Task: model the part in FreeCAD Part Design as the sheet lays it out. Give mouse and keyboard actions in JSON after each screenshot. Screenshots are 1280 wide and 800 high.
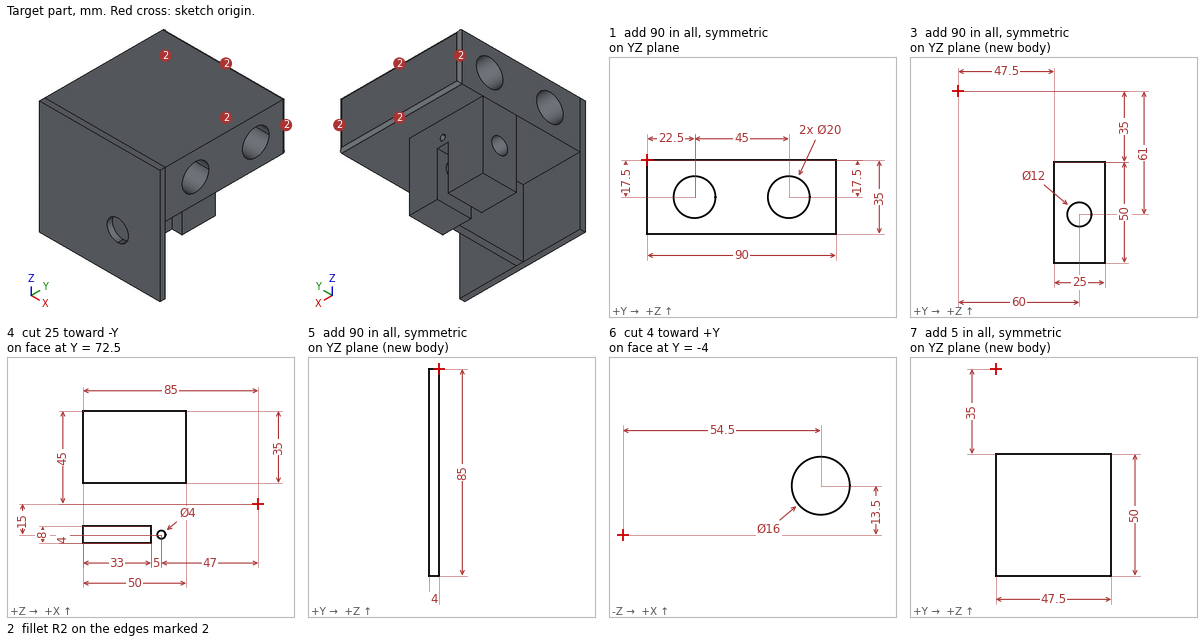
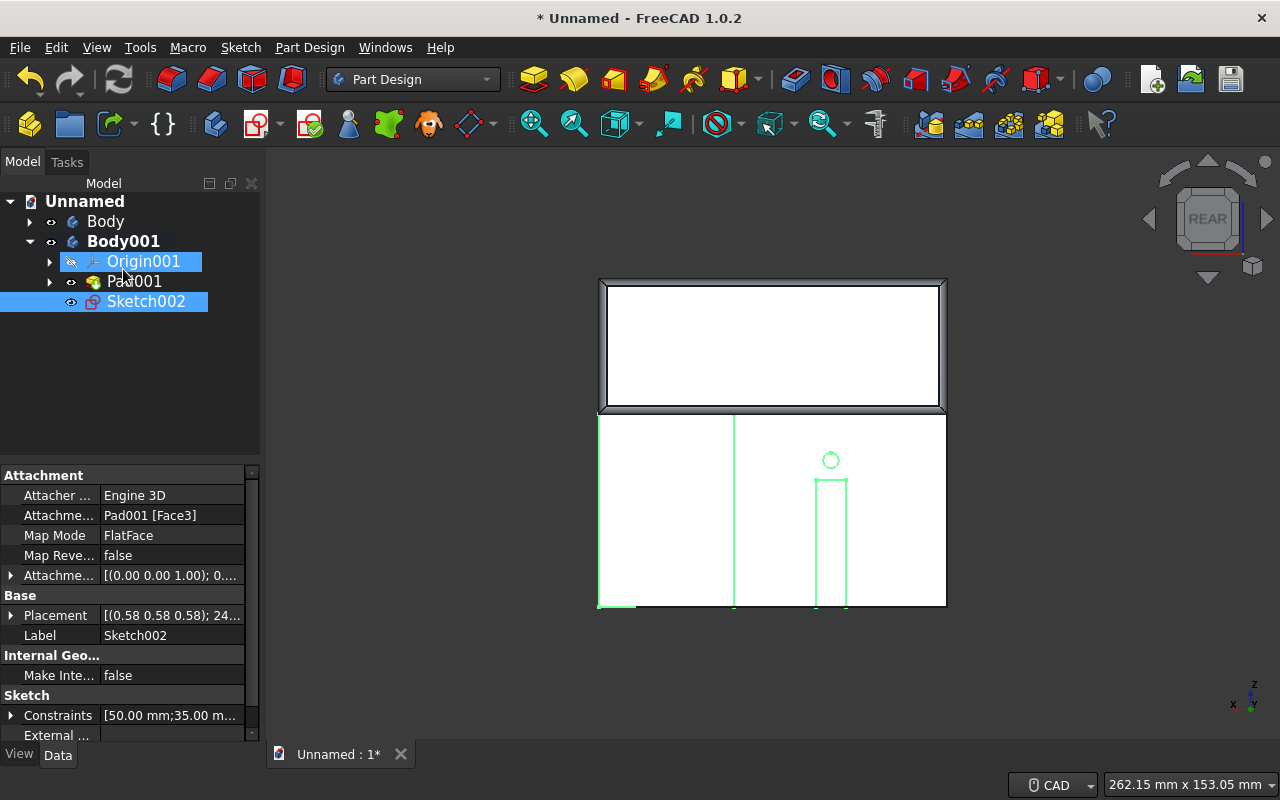
{"action": "left_click", "coordinate": [796, 80]}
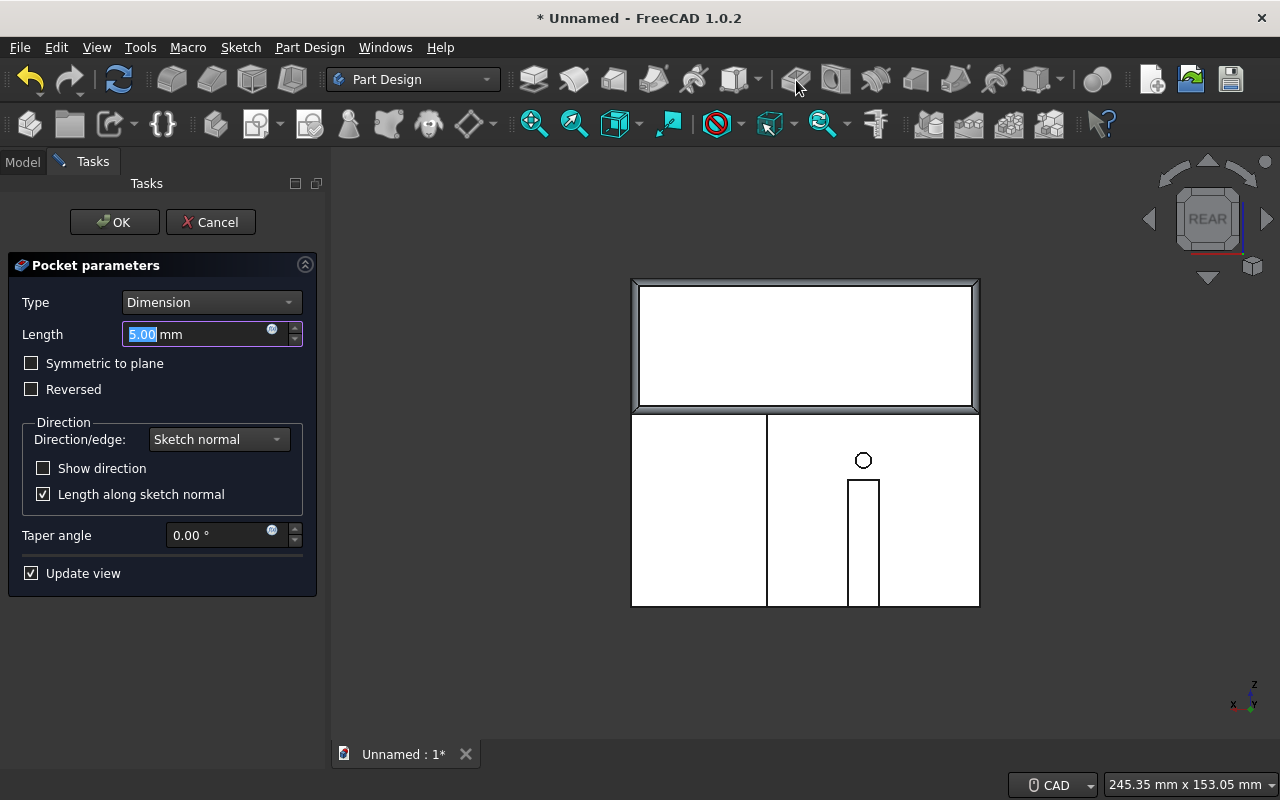
{"action": "type", "text": "25"}
{"action": "key", "text": "Tab"}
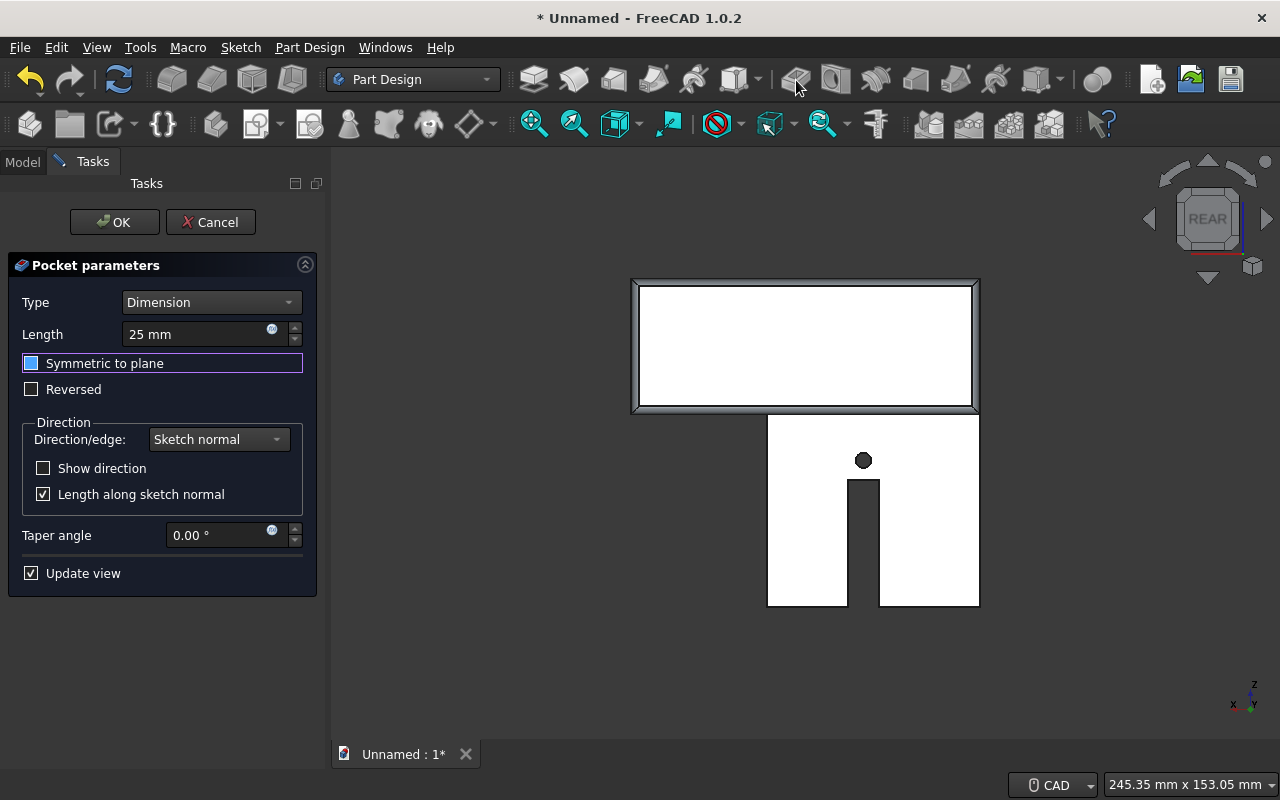
{"action": "left_click", "coordinate": [115, 222]}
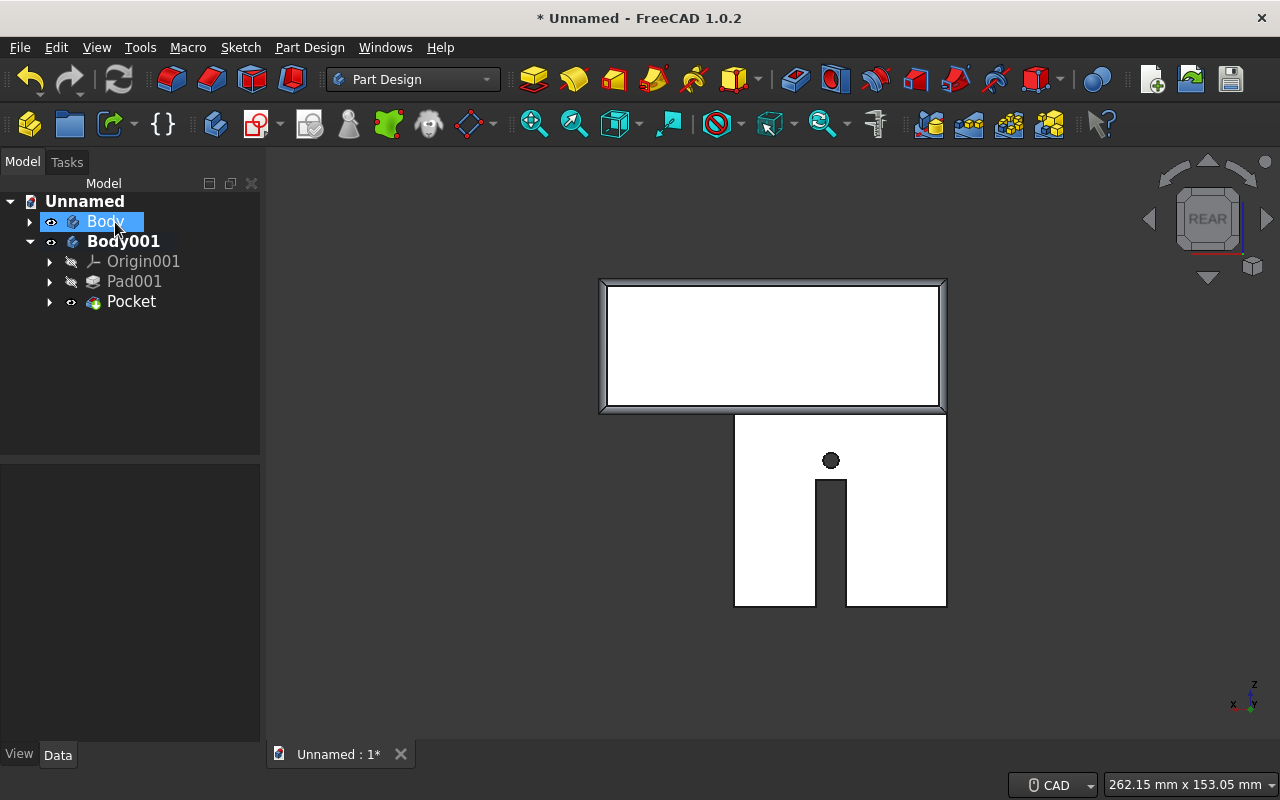
{"action": "left_click", "coordinate": [536, 124]}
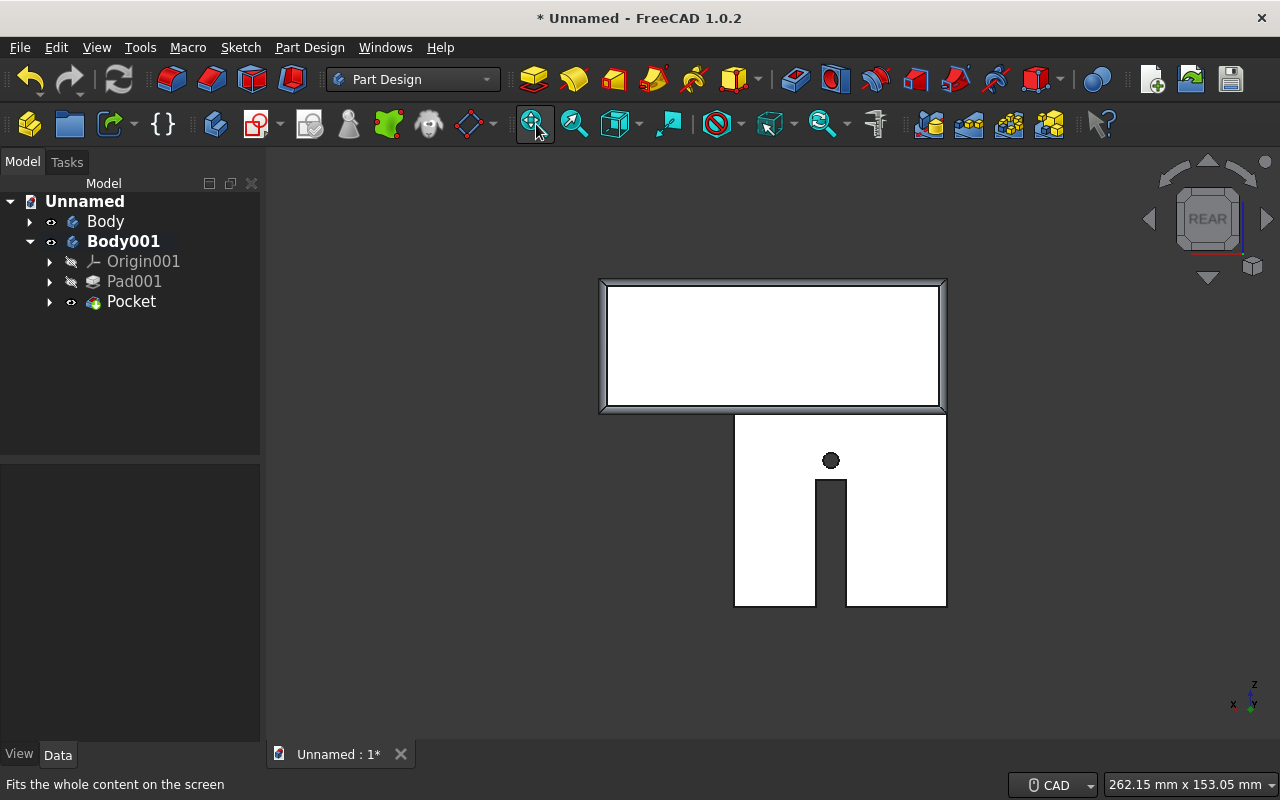
{"action": "left_click", "coordinate": [216, 124]}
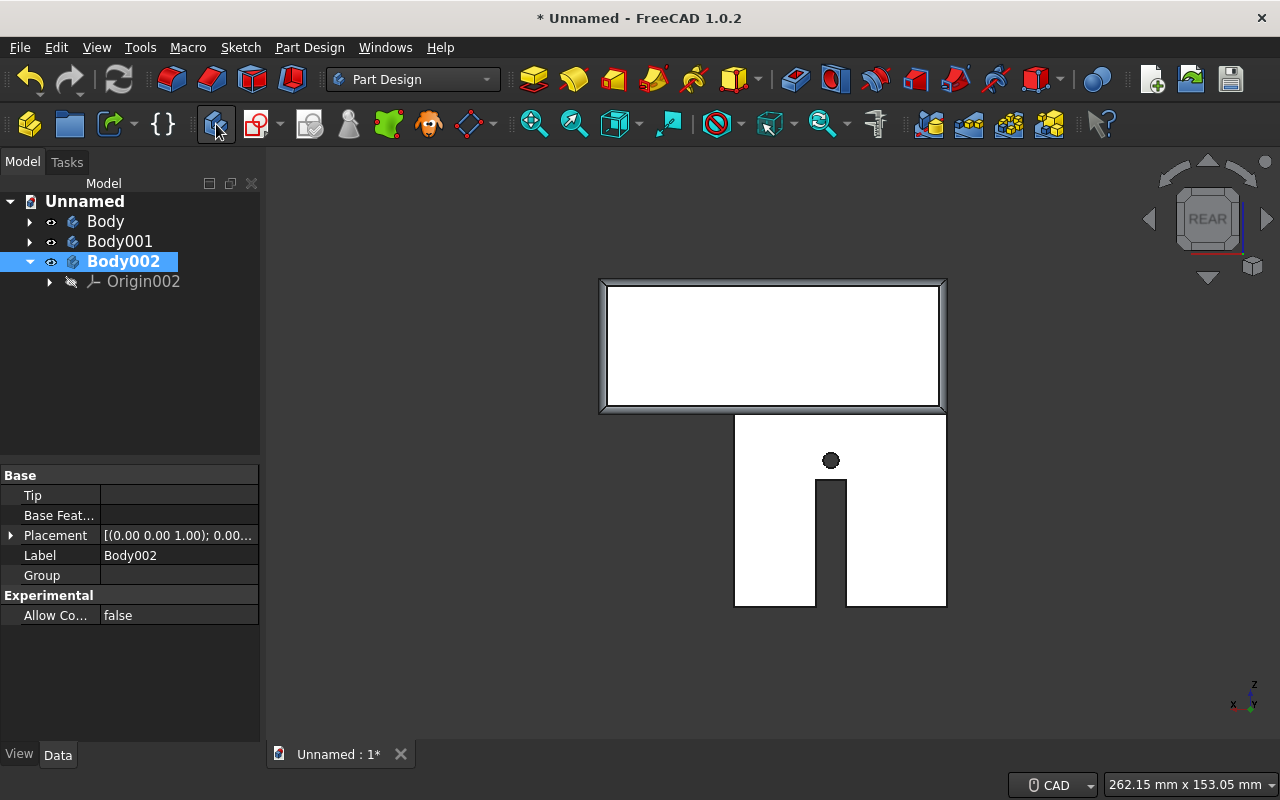
{"action": "left_click", "coordinate": [306, 699]}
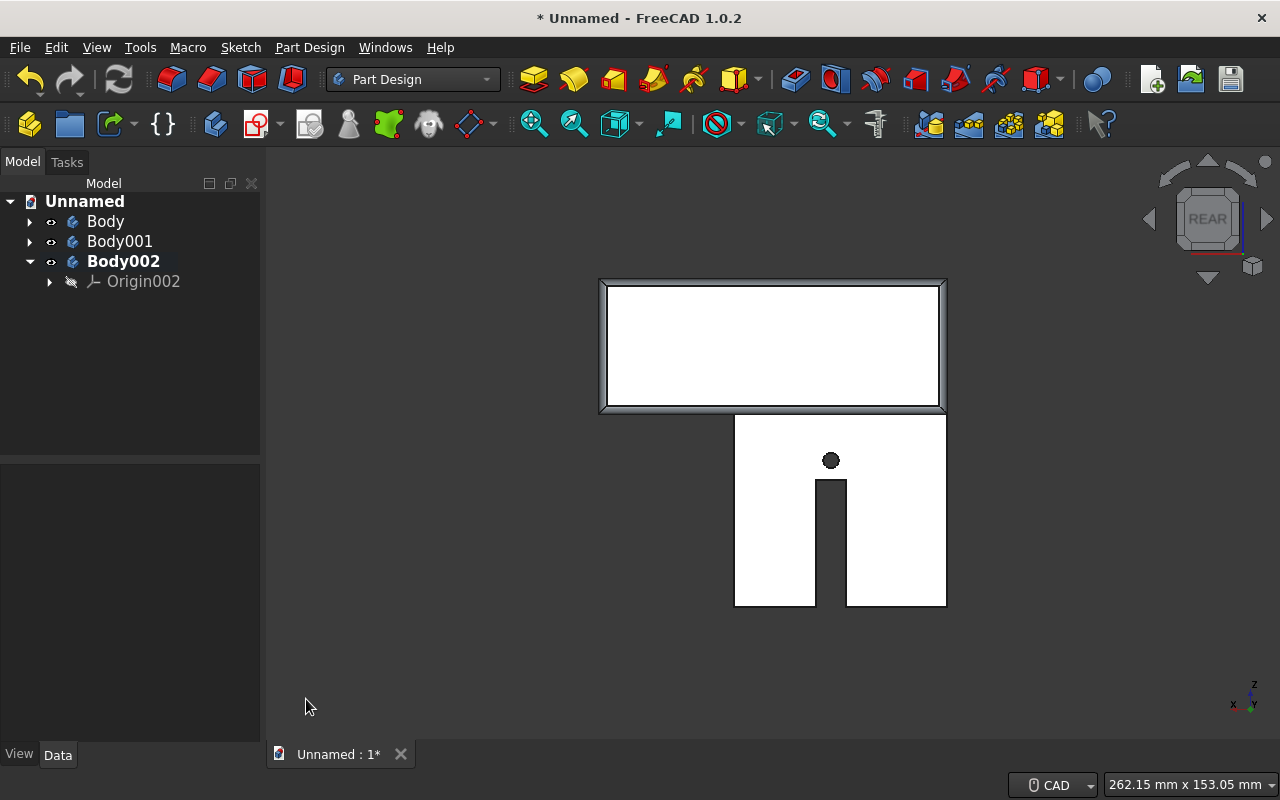
{"action": "left_click", "coordinate": [256, 124]}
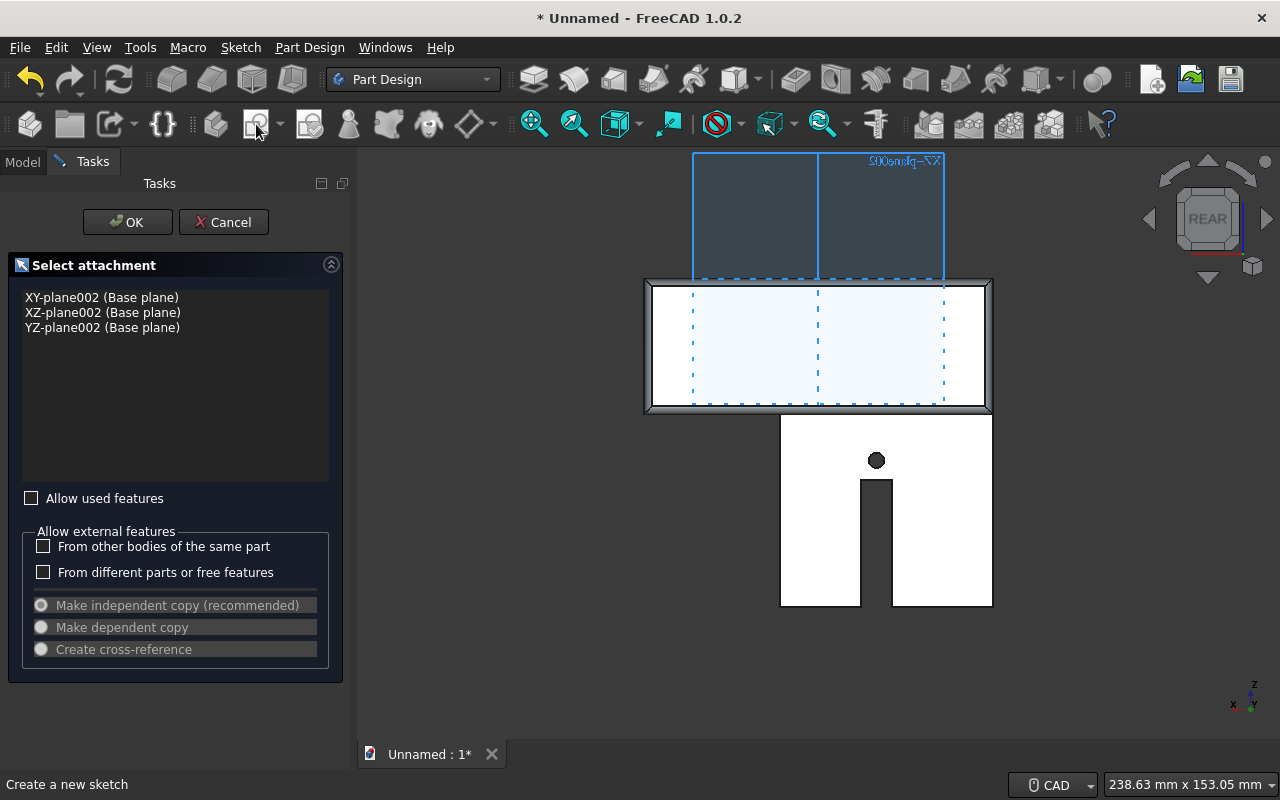
{"action": "left_click", "coordinate": [82, 328]}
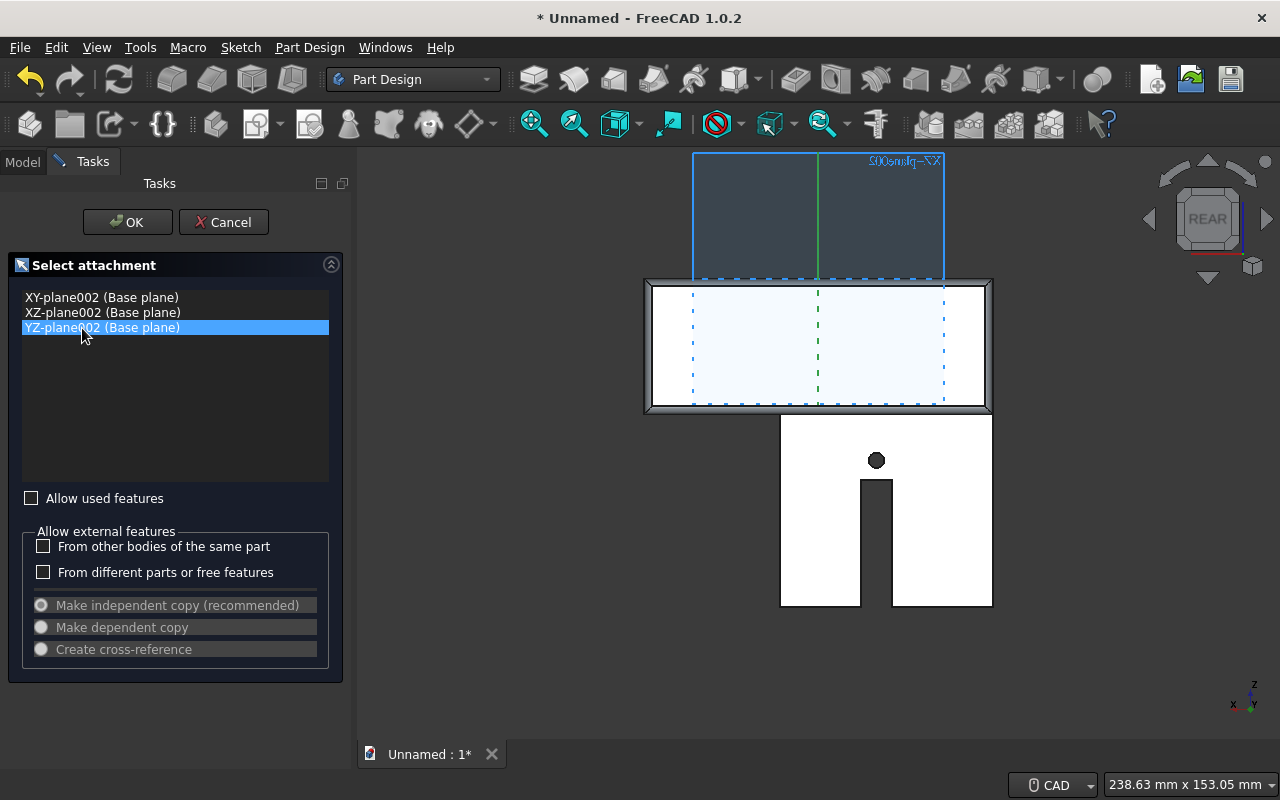
{"action": "left_click", "coordinate": [128, 222]}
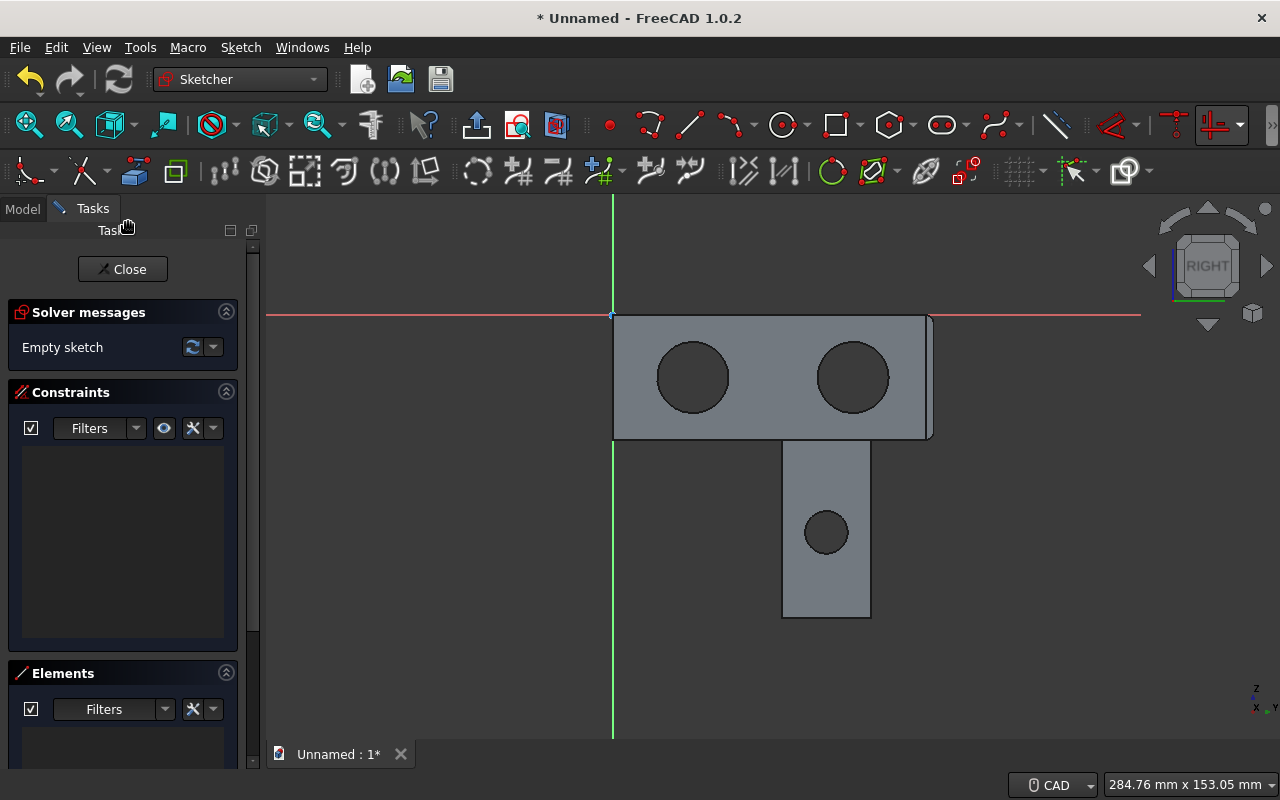
{"action": "key", "text": "g r"}